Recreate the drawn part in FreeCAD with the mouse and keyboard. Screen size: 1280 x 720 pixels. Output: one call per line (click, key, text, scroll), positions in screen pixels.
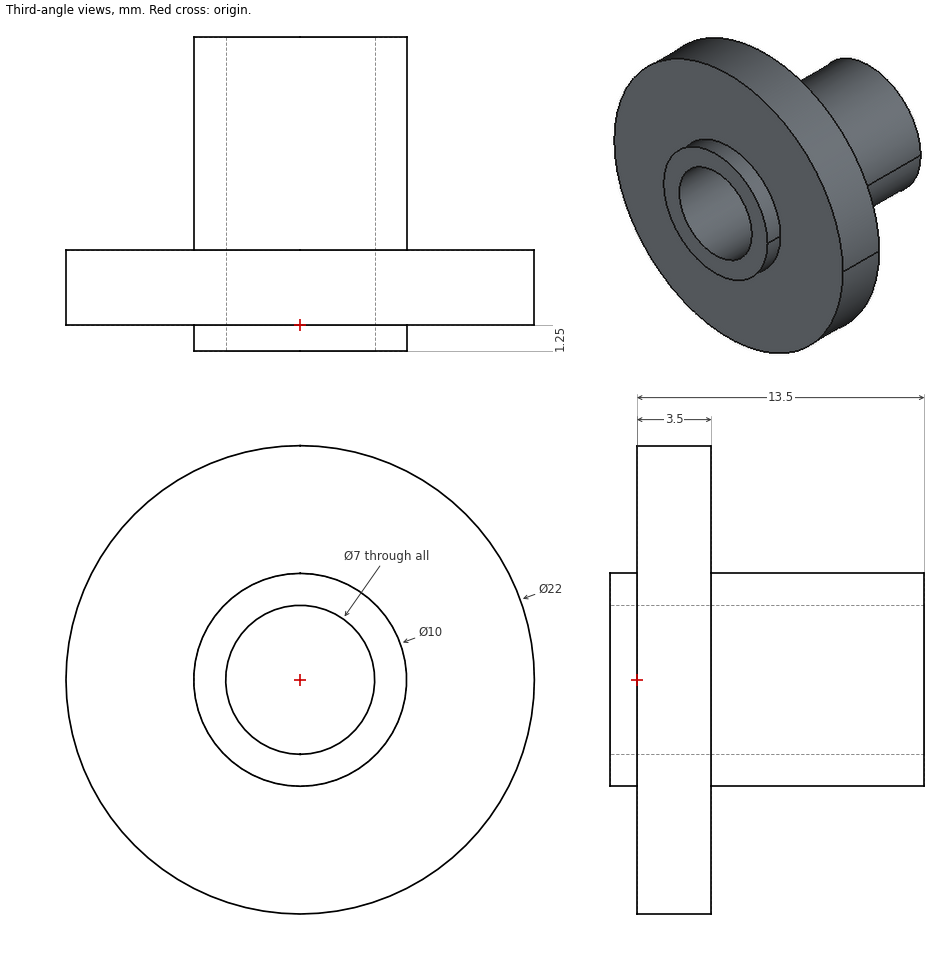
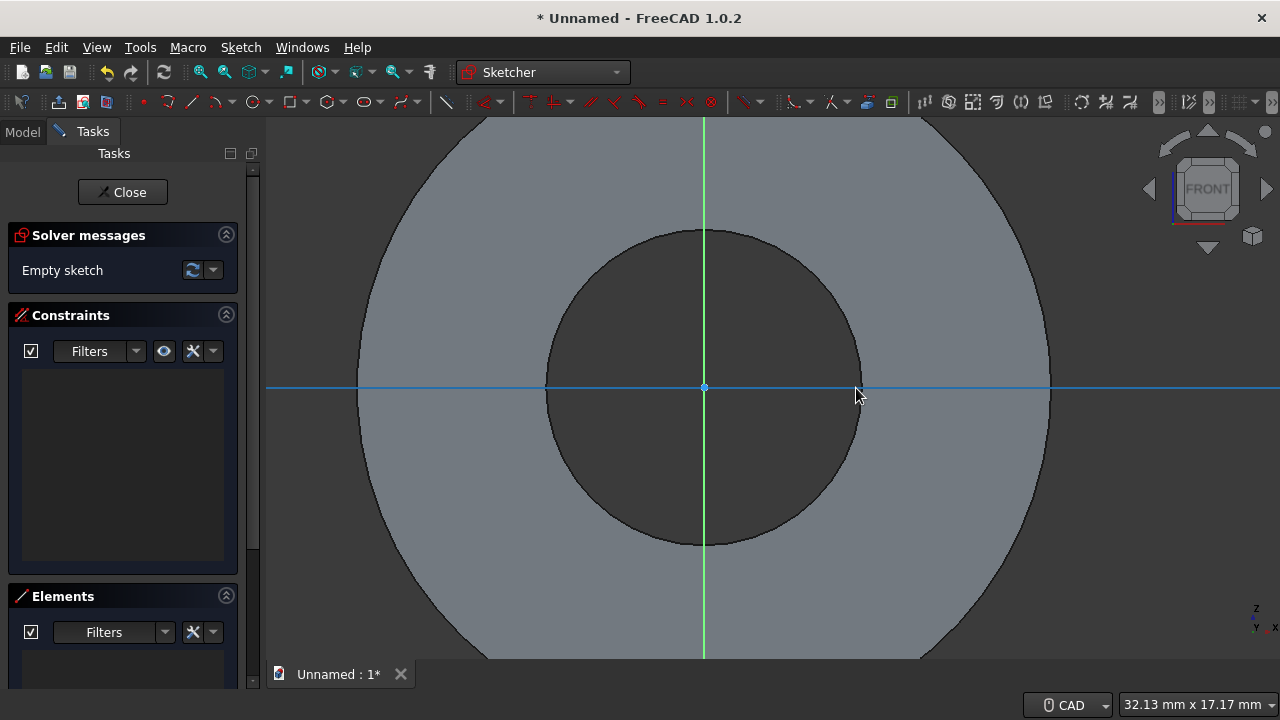
key(g)
key(c)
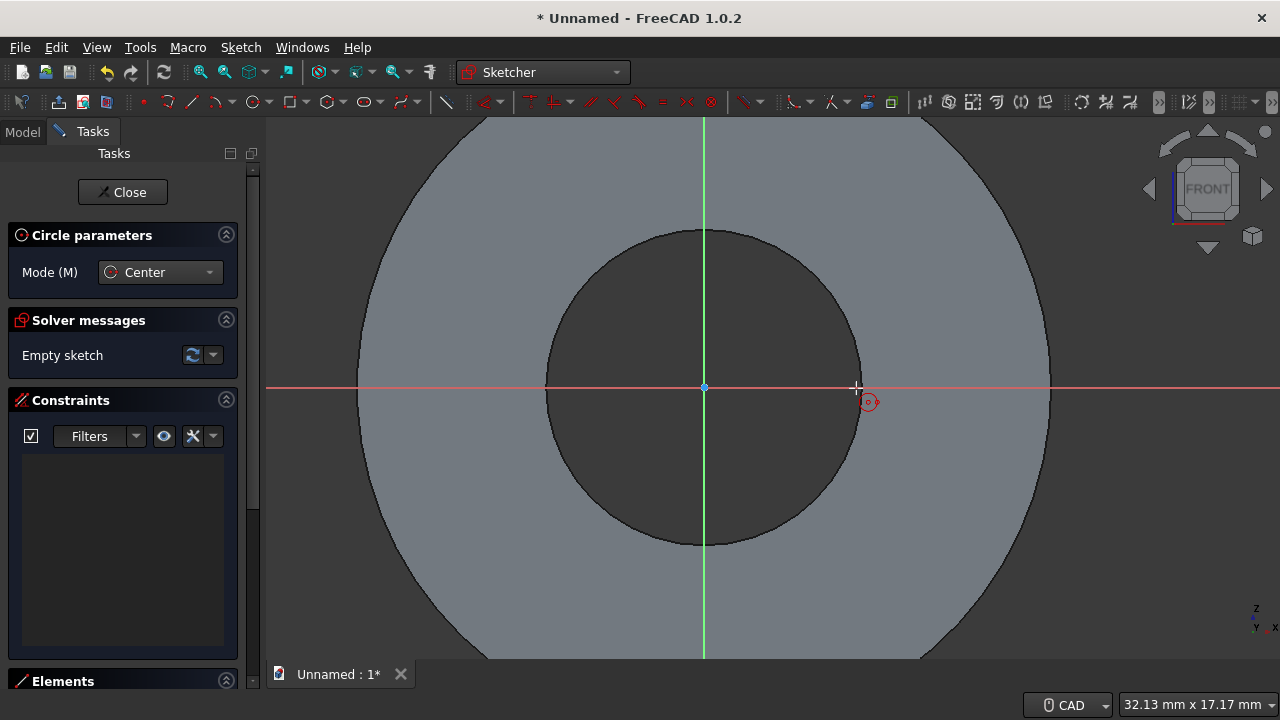
click(704, 388)
move(816, 276)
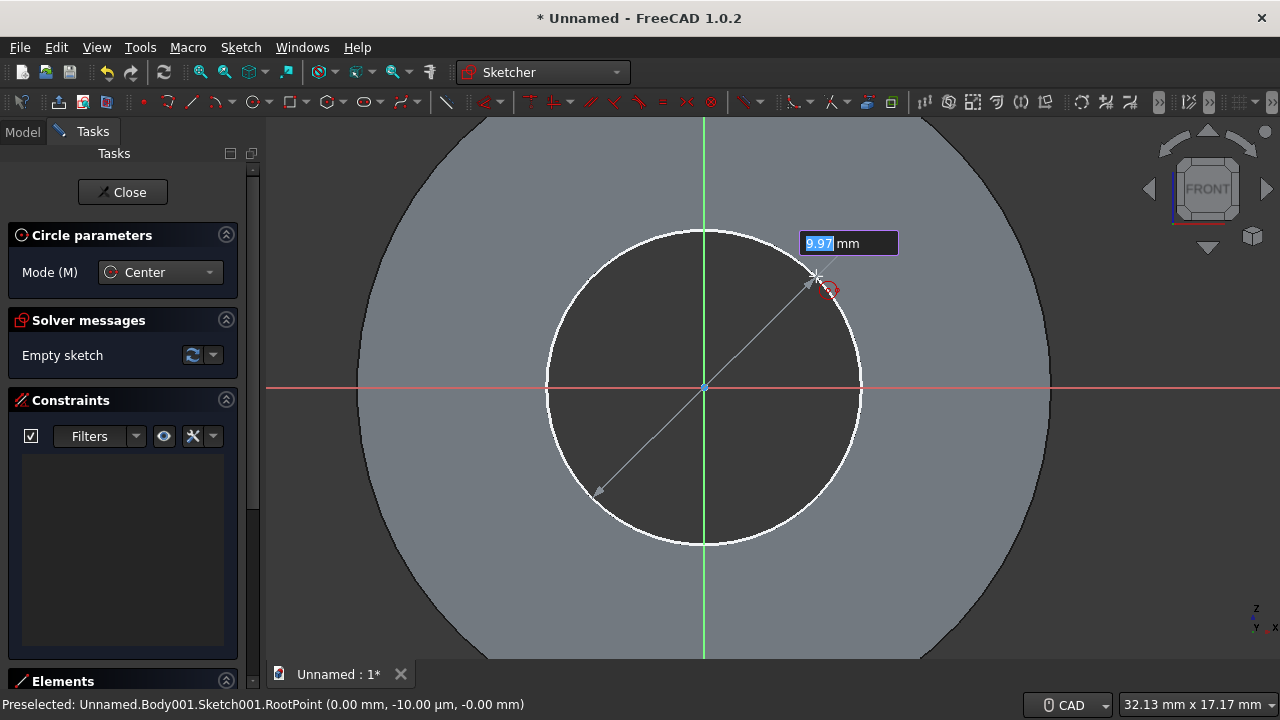
text(10)
key(Return)
key(Escape)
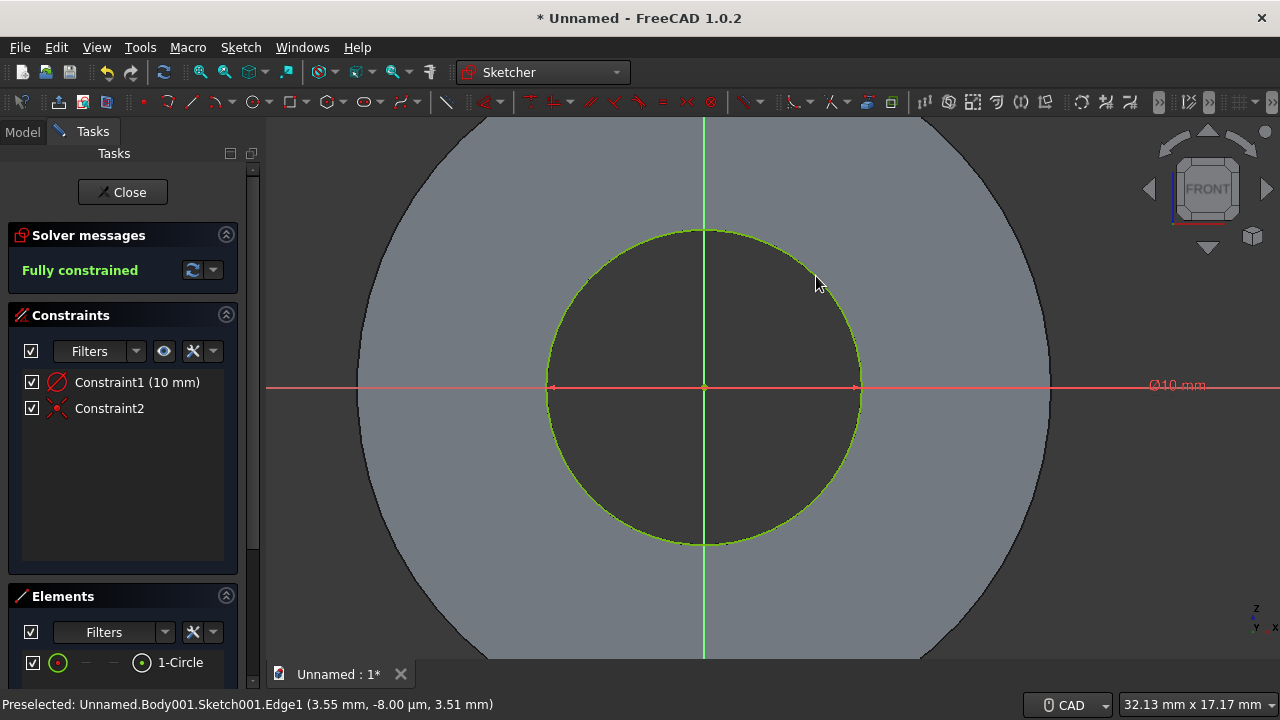
click(123, 192)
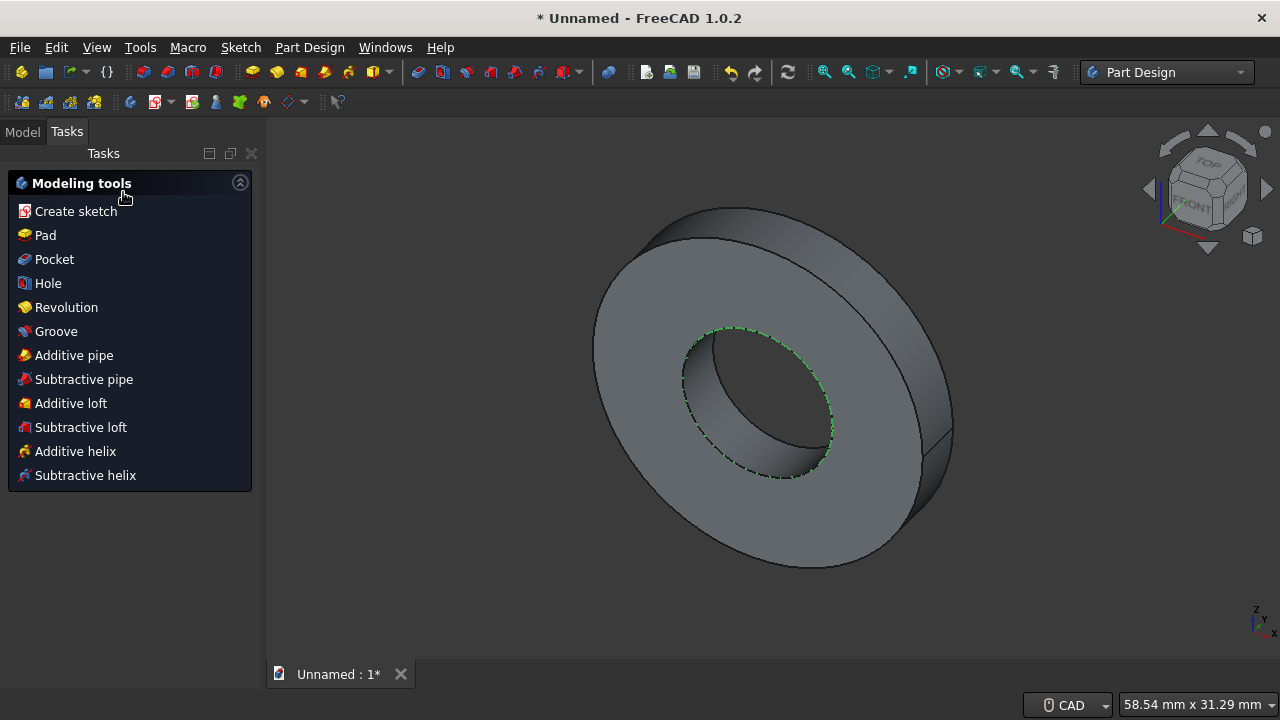
click(254, 72)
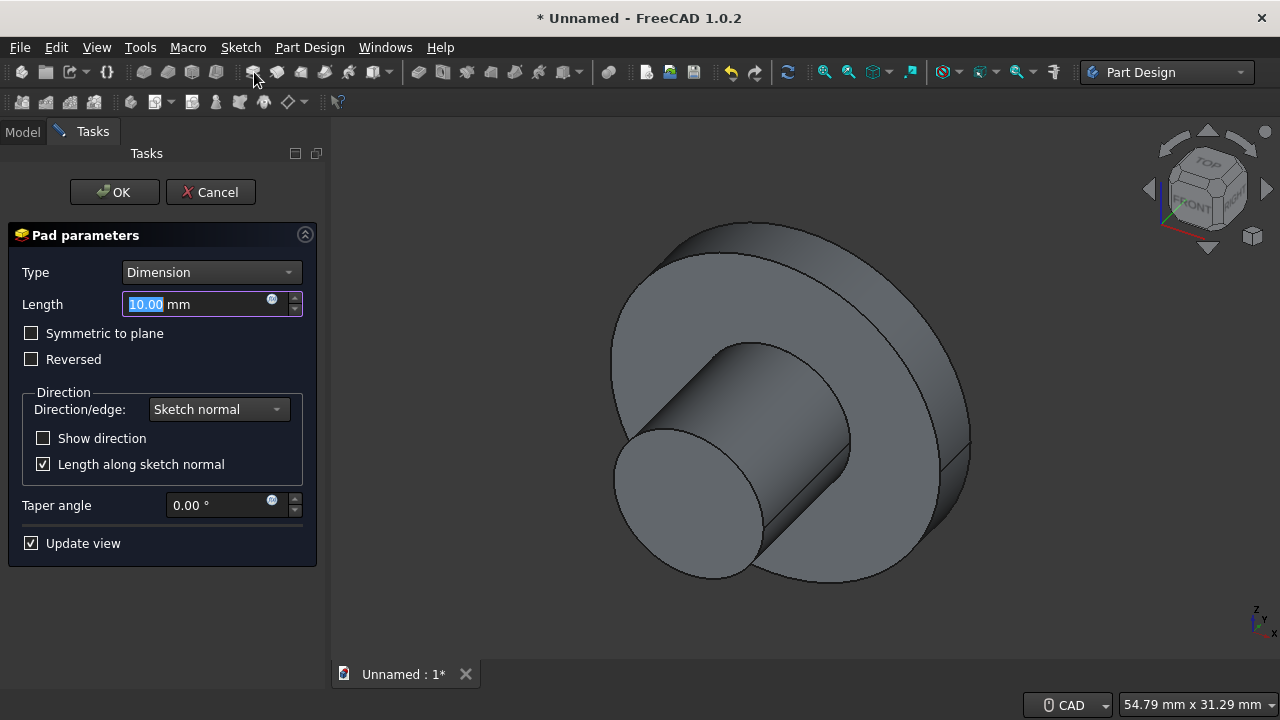
text(1.25)
key(Tab)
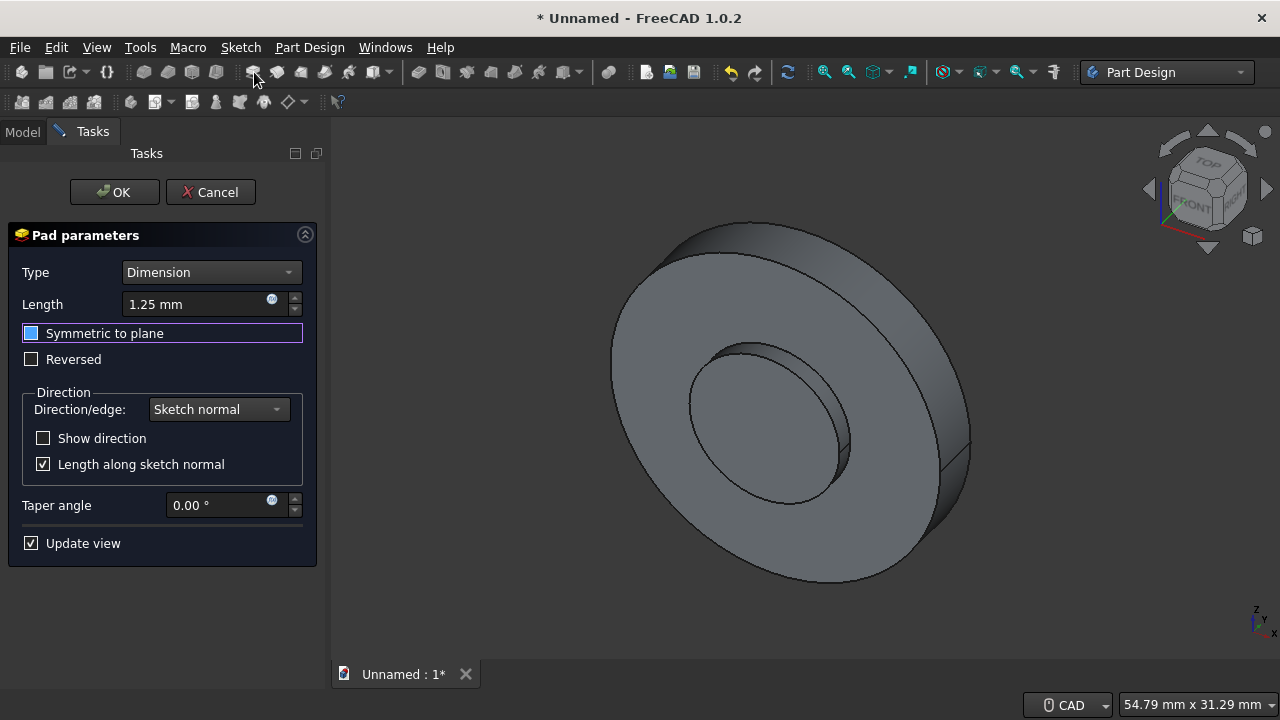
click(115, 192)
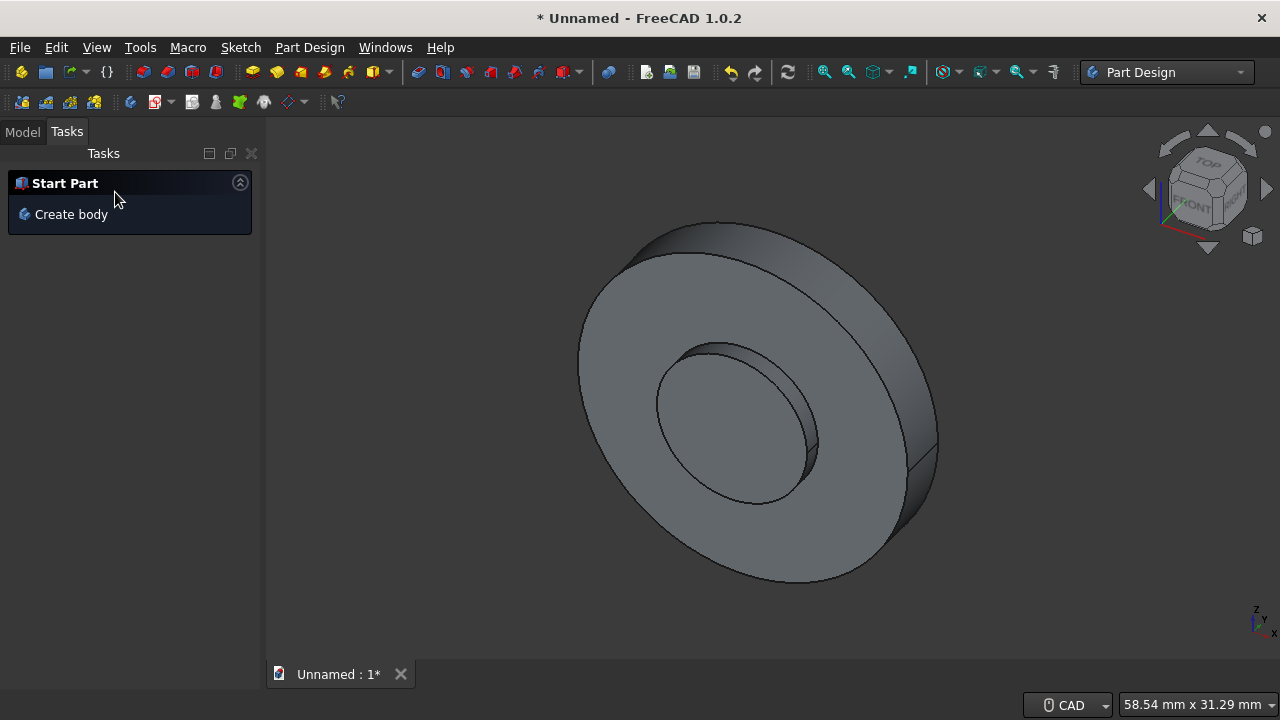
click(826, 72)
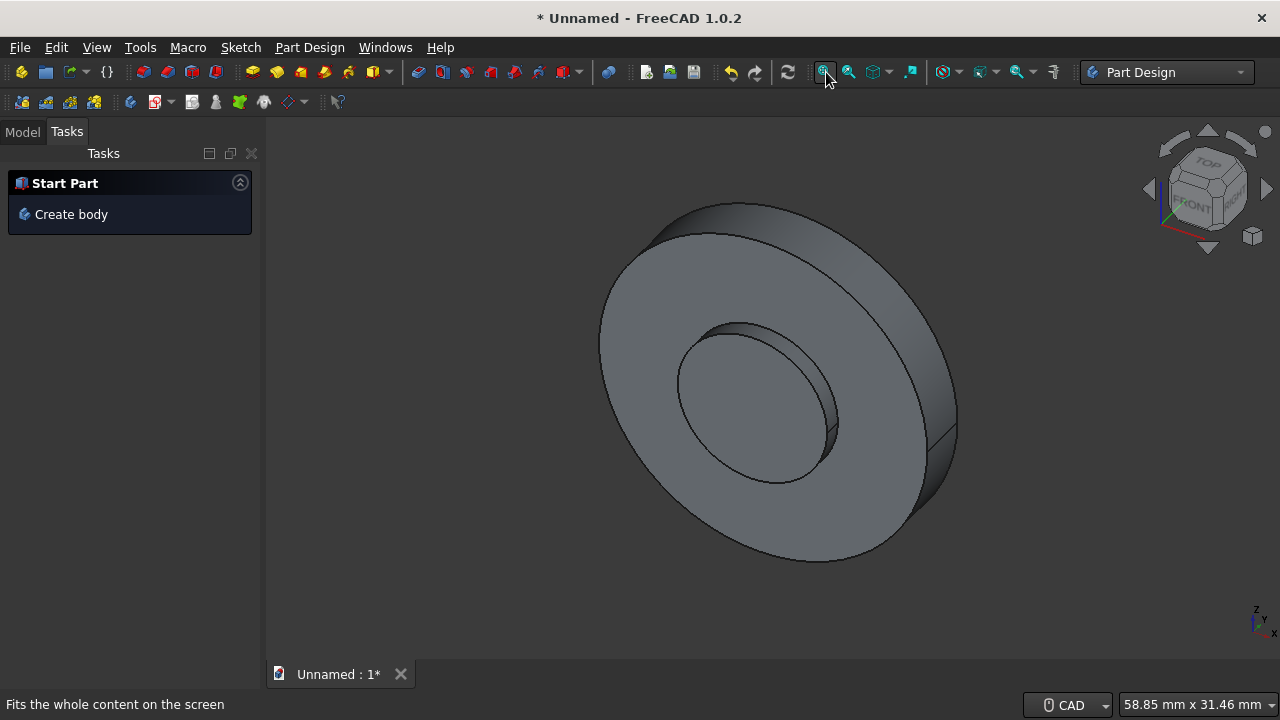
click(23, 131)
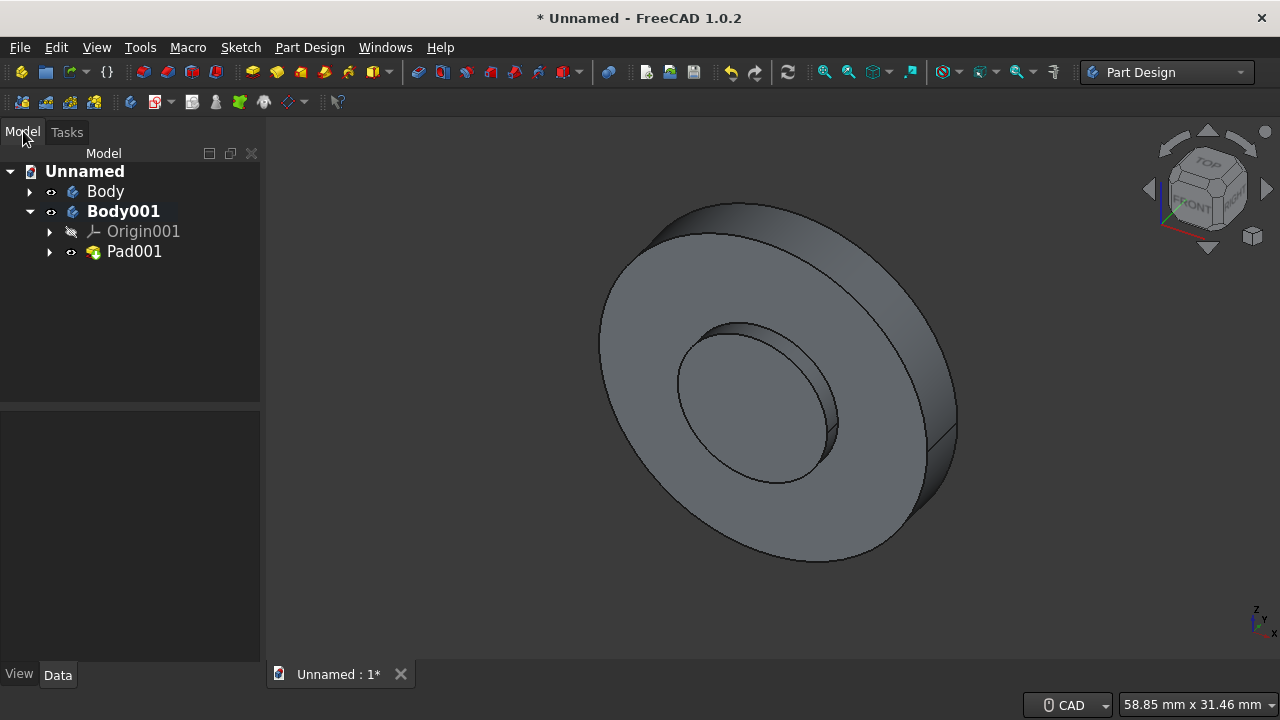
double_click(96, 192)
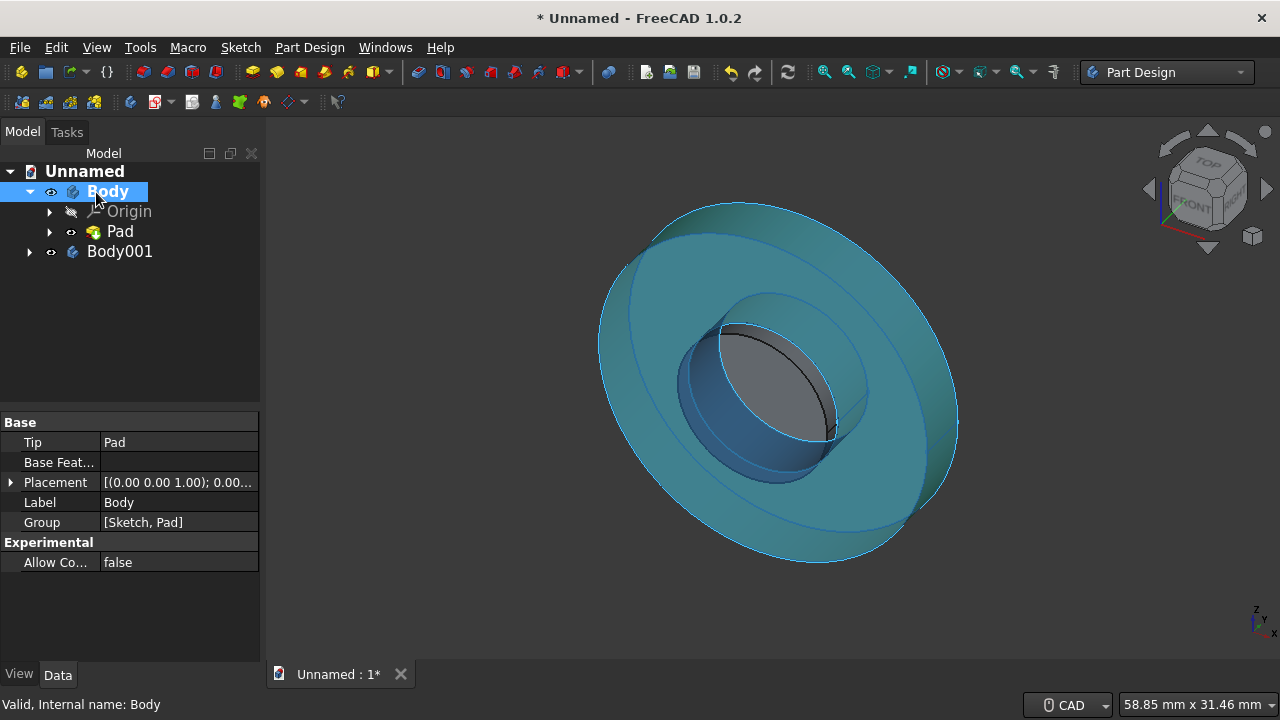
click(96, 192)